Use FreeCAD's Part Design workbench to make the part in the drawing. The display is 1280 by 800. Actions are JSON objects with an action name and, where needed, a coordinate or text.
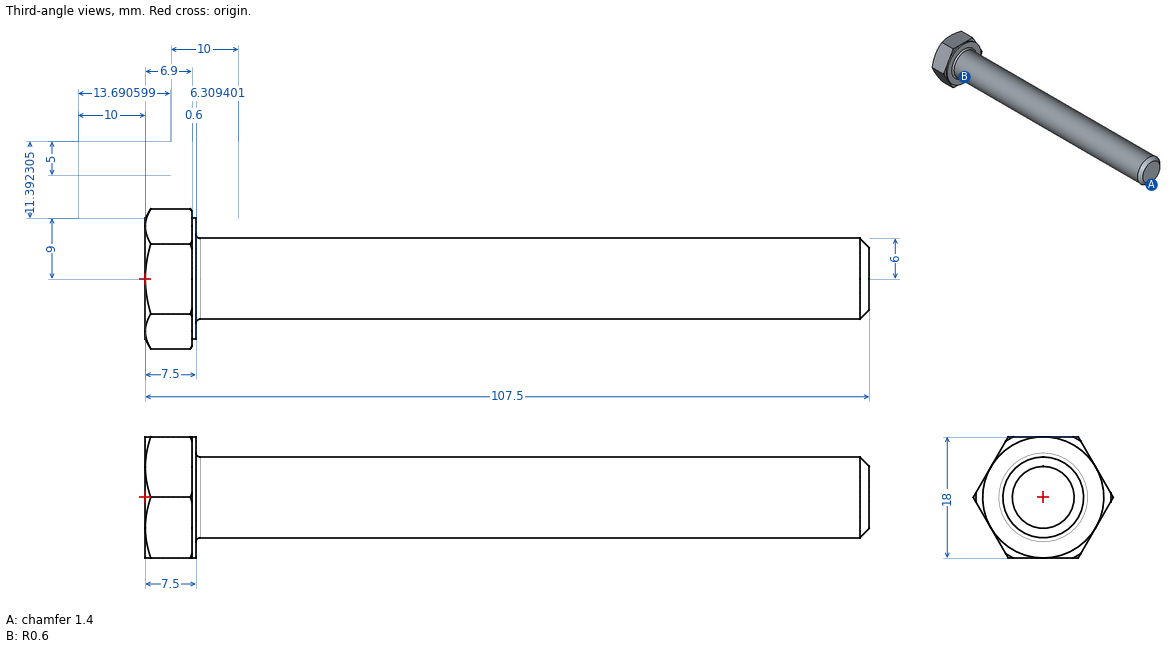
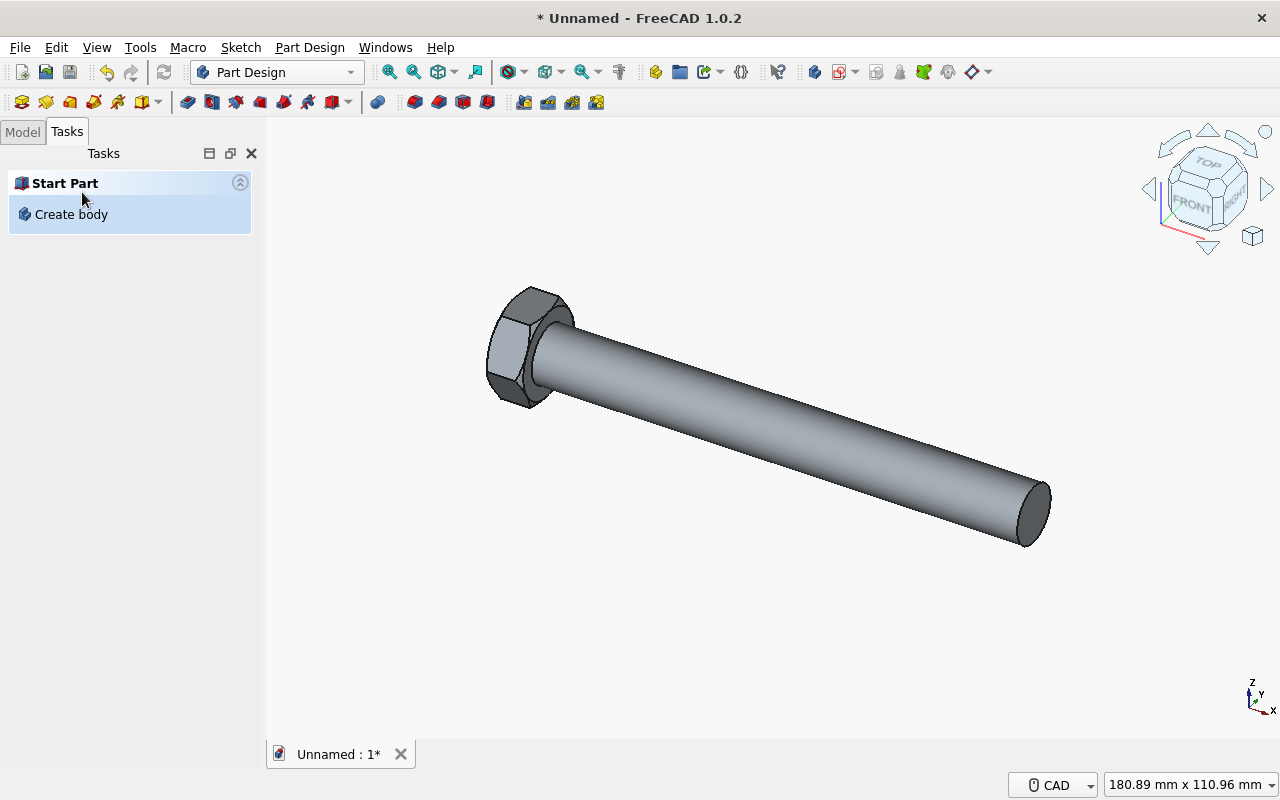
{"action": "left_click", "coordinate": [840, 72]}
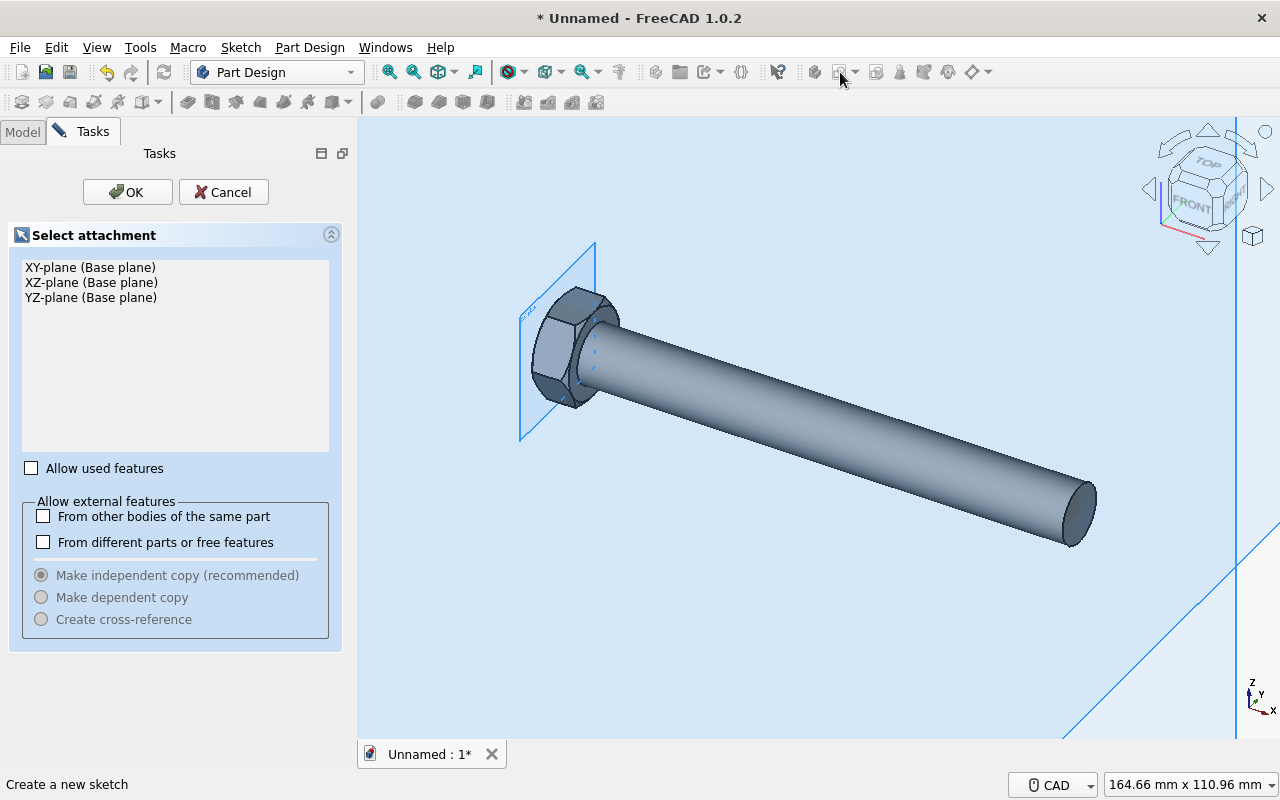
{"action": "left_click", "coordinate": [82, 268]}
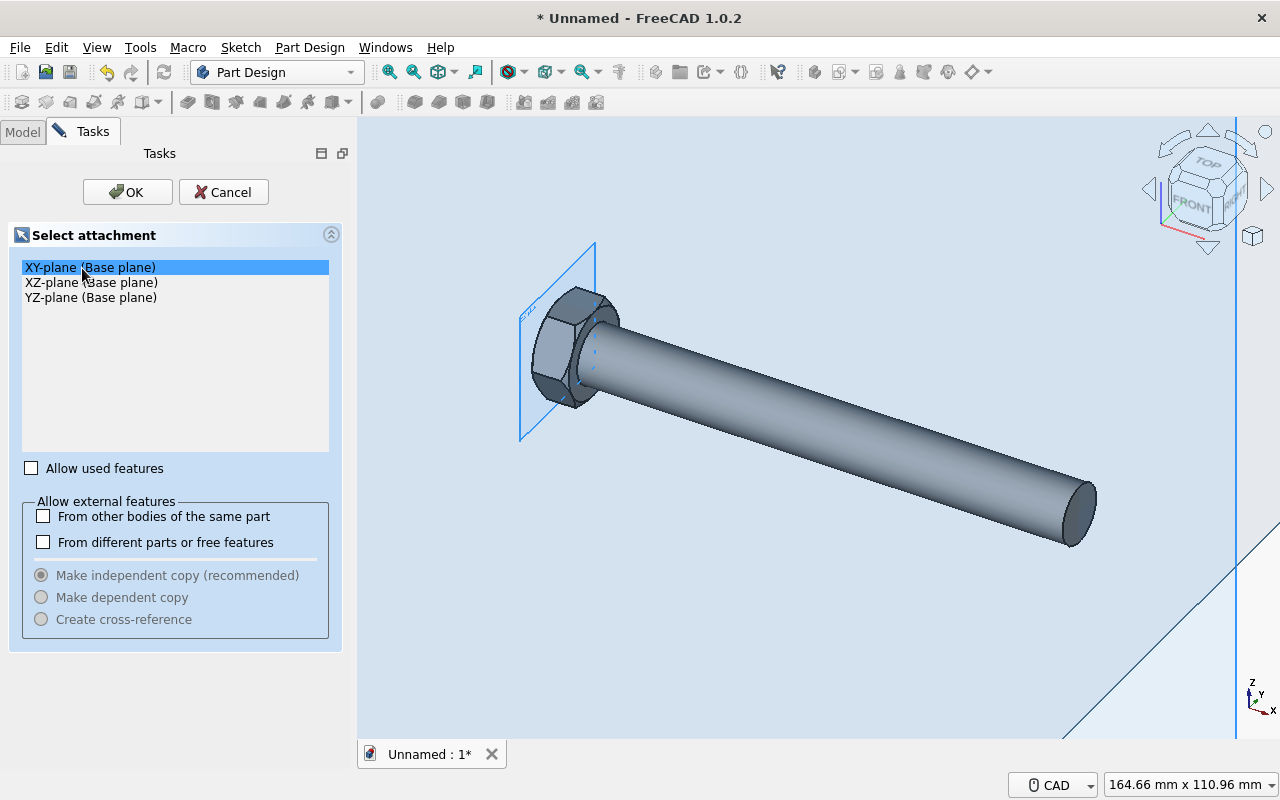
{"action": "left_click", "coordinate": [128, 192]}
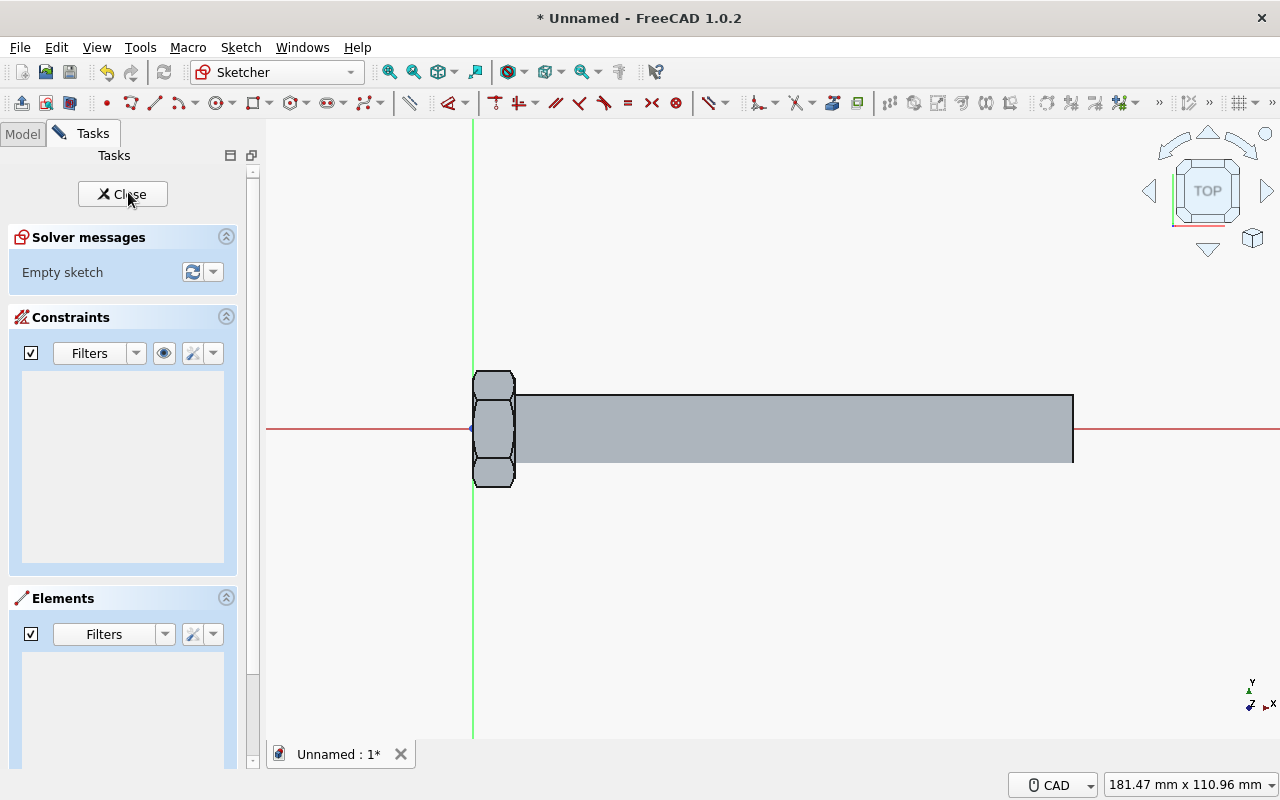
{"action": "key", "text": "q s"}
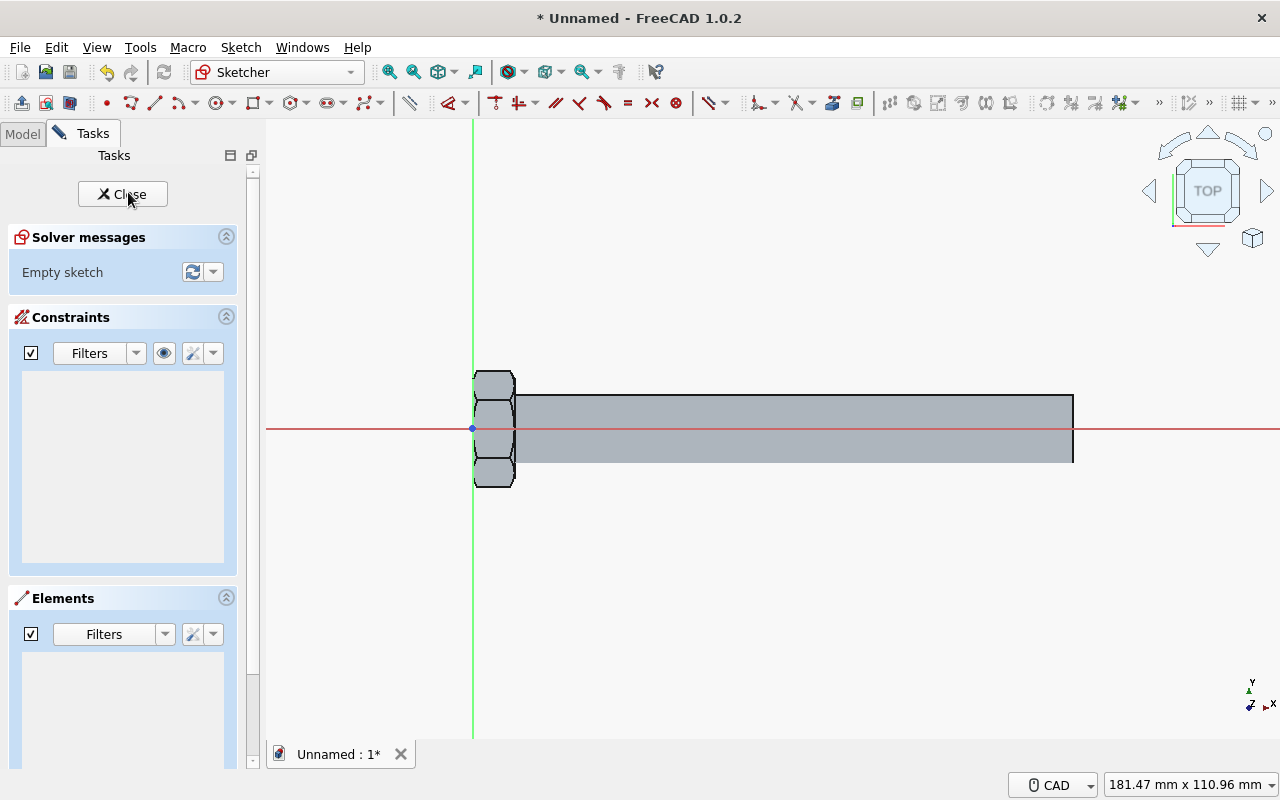
{"action": "scroll", "coordinate": [403, 347], "scroll_direction": "up", "scroll_amount": 6}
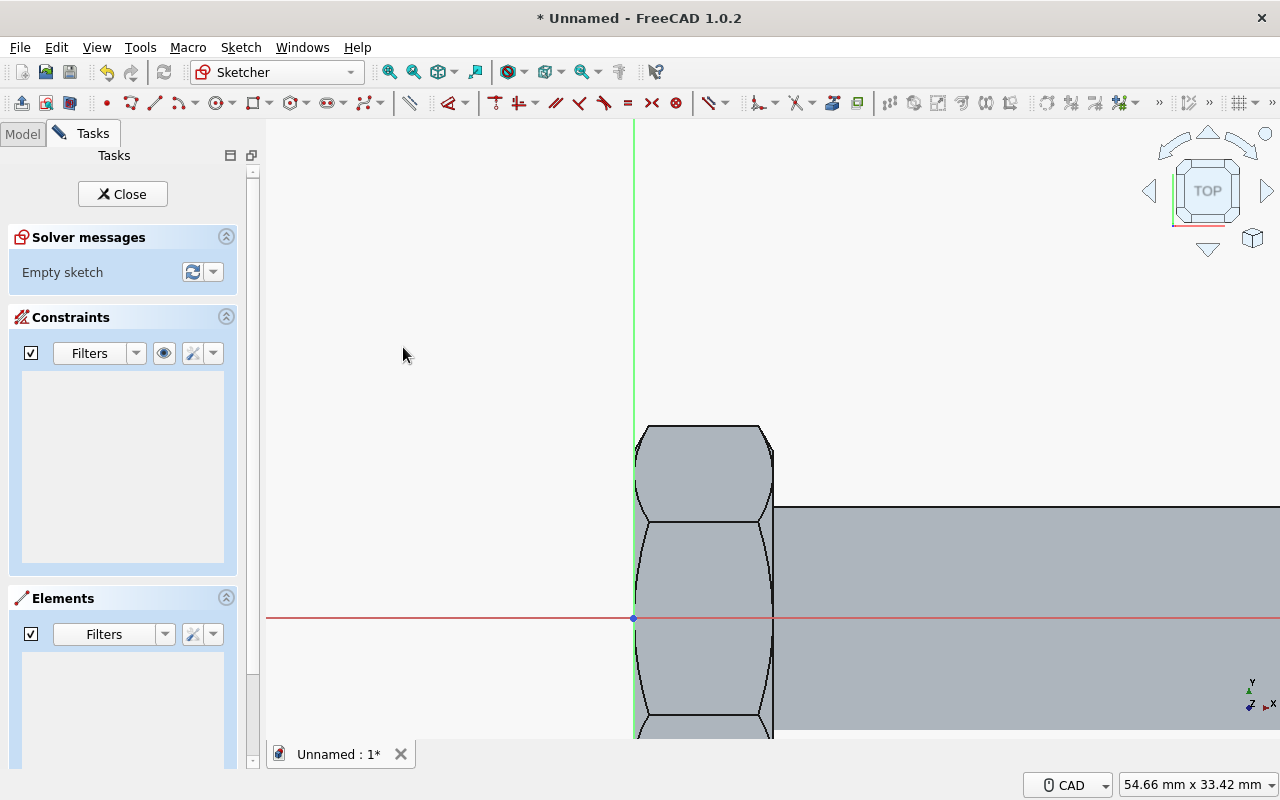
{"action": "left_click", "coordinate": [254, 104]}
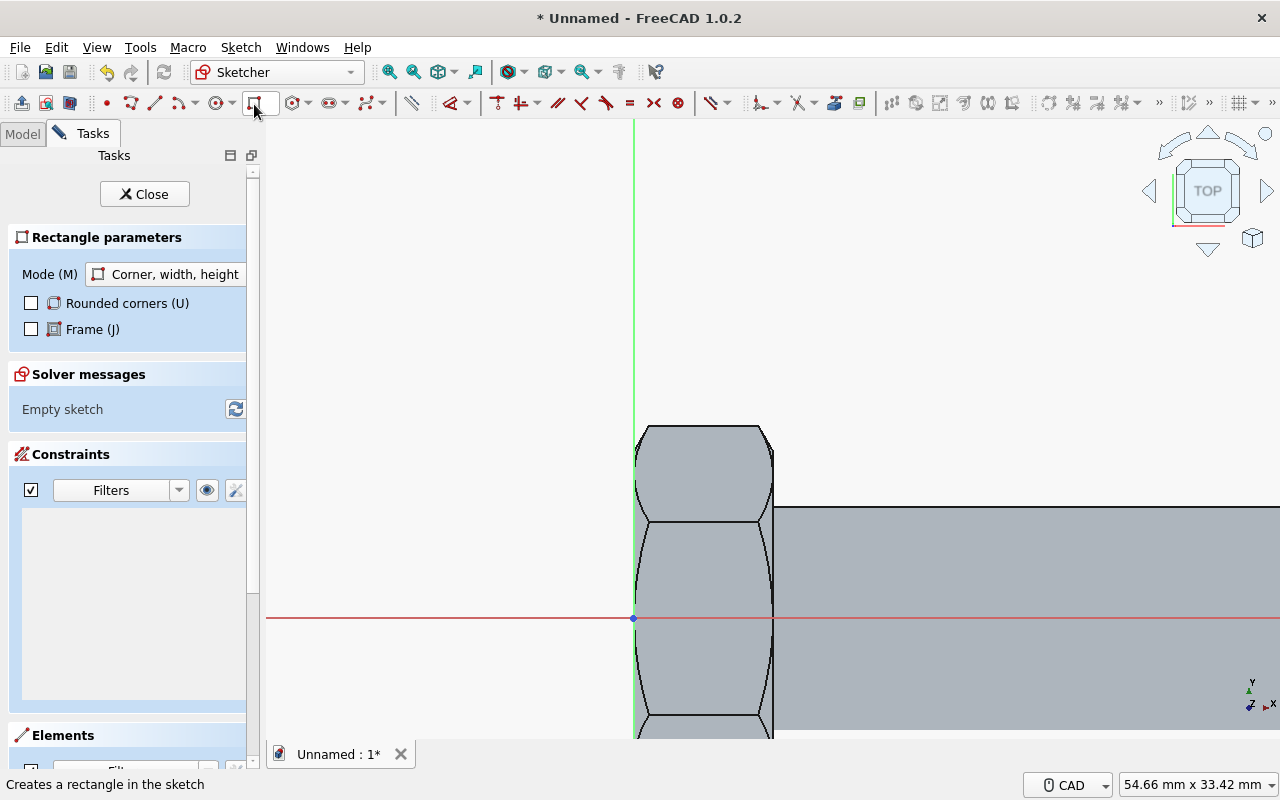
{"action": "scroll", "coordinate": [762, 240], "scroll_direction": "up", "scroll_amount": 2}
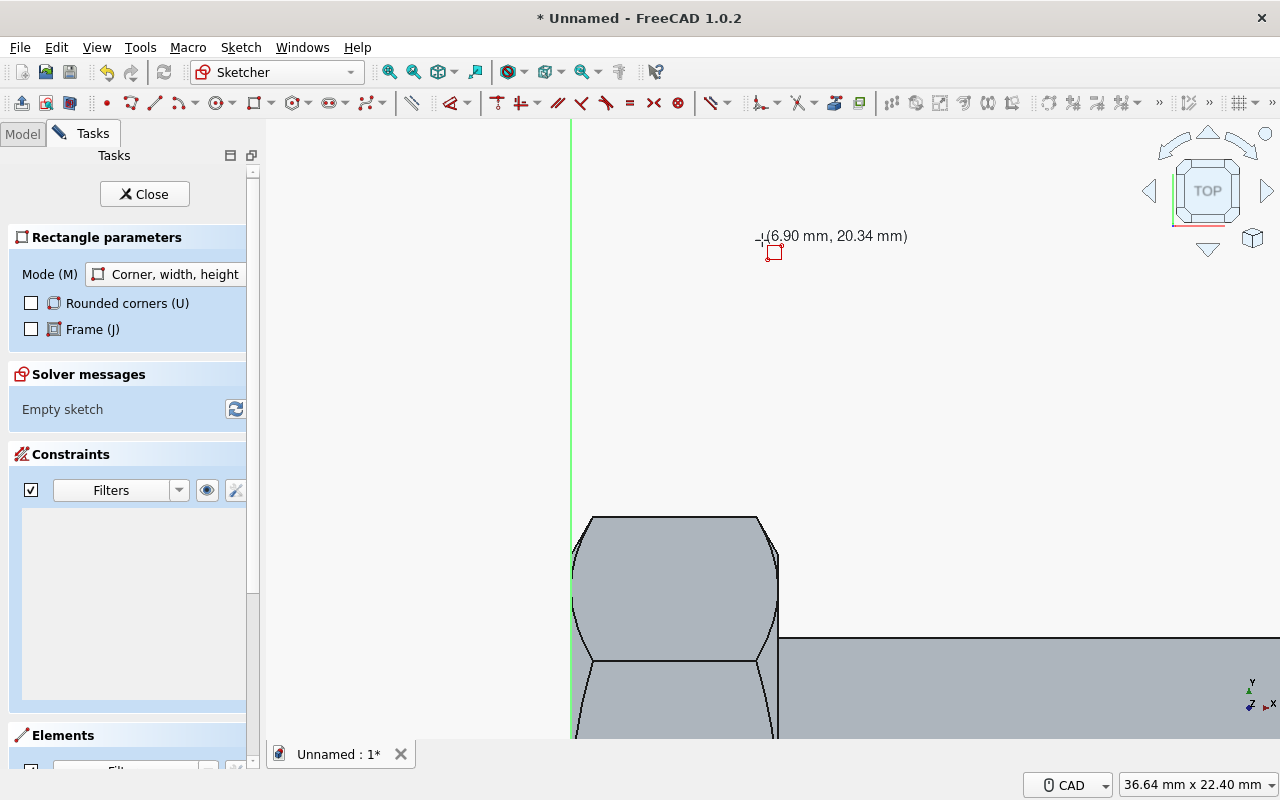
{"action": "left_click", "coordinate": [762, 240]}
{"action": "mouse_move", "coordinate": [778, 555]}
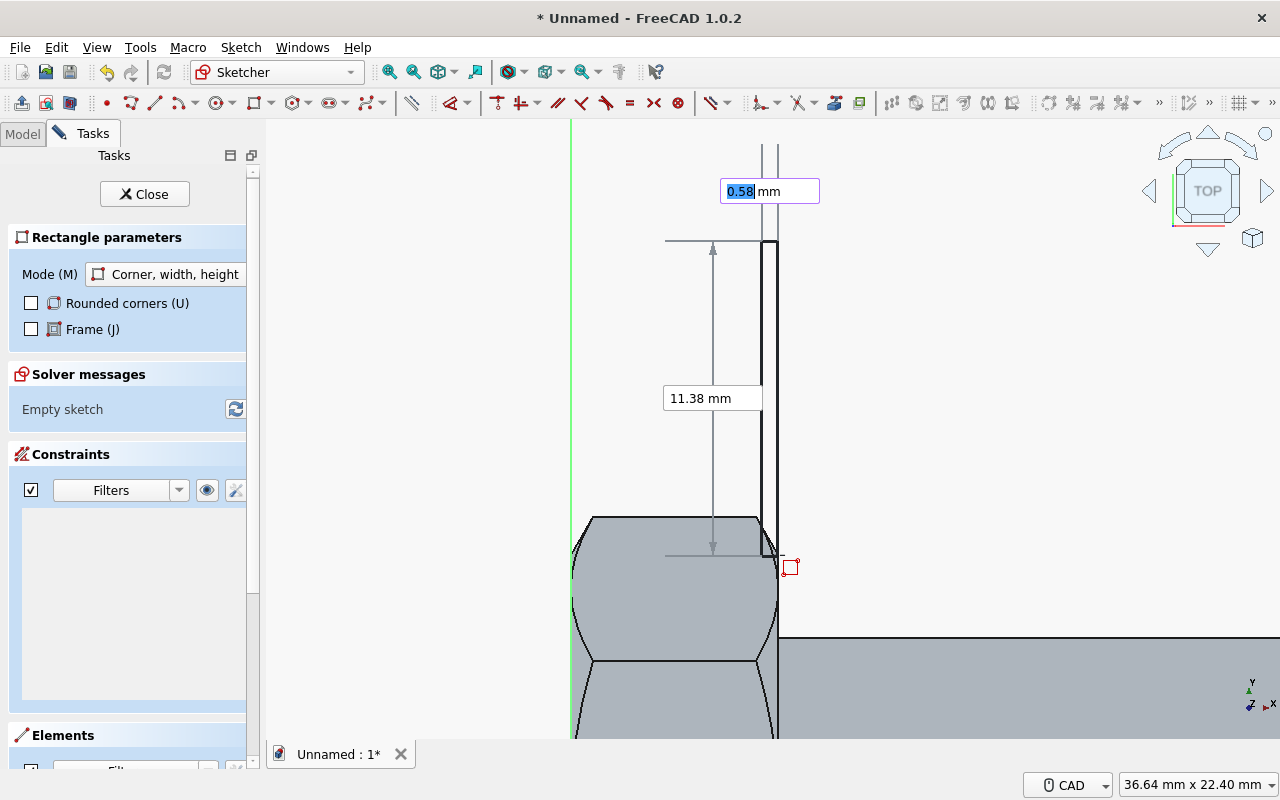
{"action": "type", "text": "0.6"}
{"action": "key", "text": "Tab"}
{"action": "type", "text": "11.392305"}
{"action": "key", "text": "Return"}
{"action": "key", "text": "Escape"}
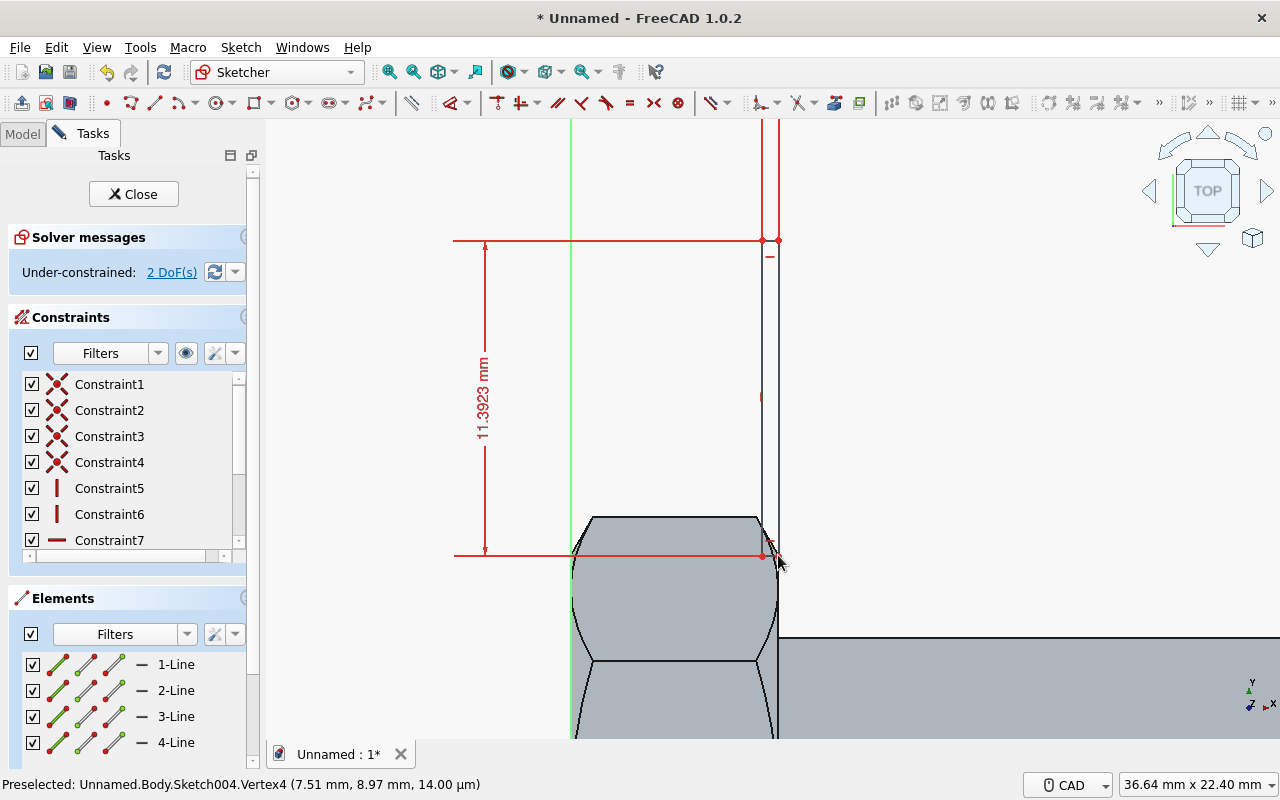
{"action": "left_click", "coordinate": [450, 104]}